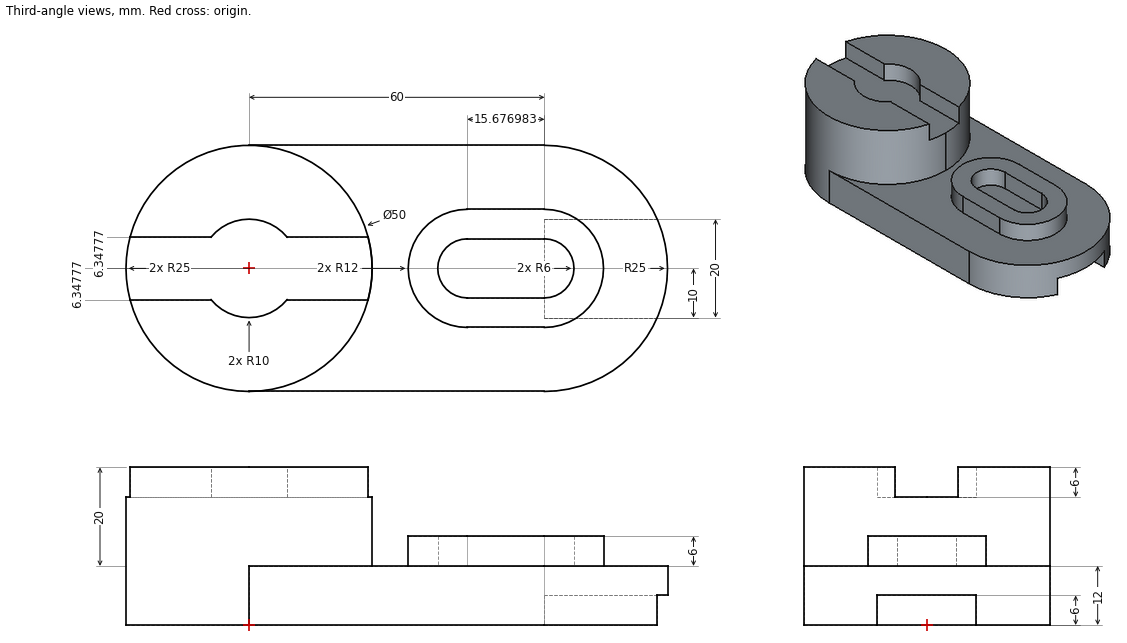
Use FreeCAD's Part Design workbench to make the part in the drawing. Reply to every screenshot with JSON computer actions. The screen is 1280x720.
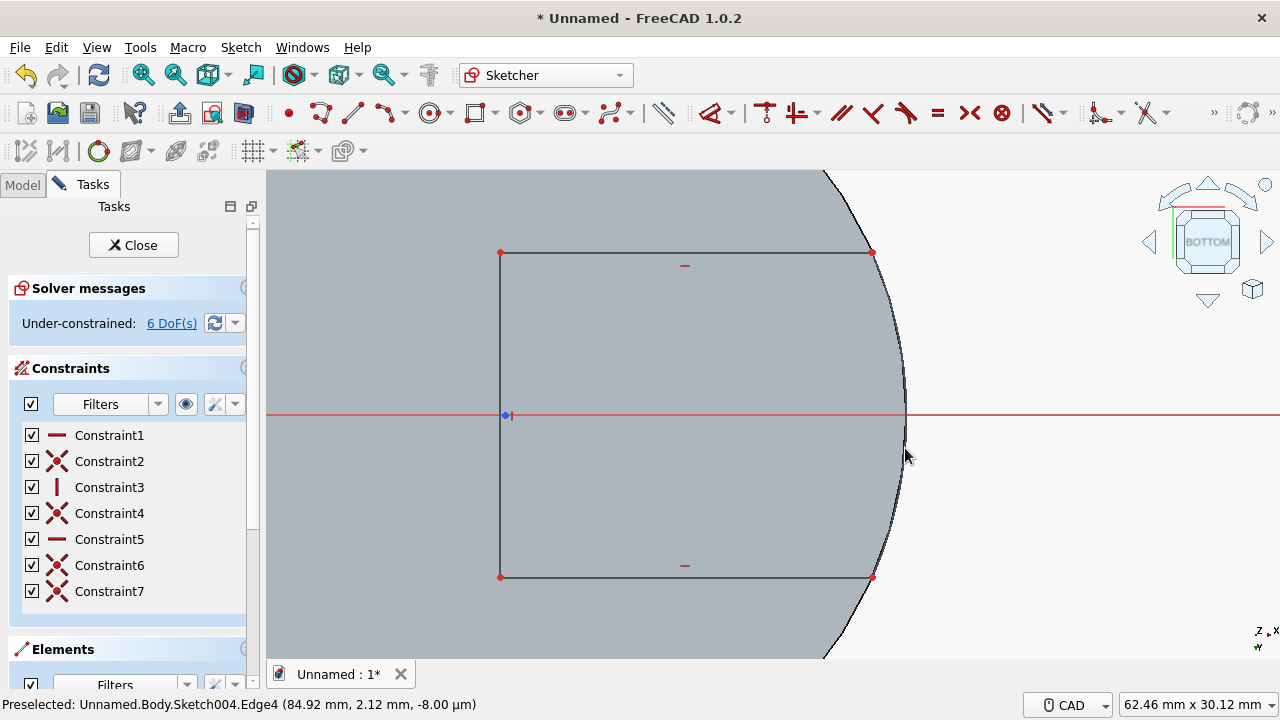
{"action": "left_click", "coordinate": [505, 416]}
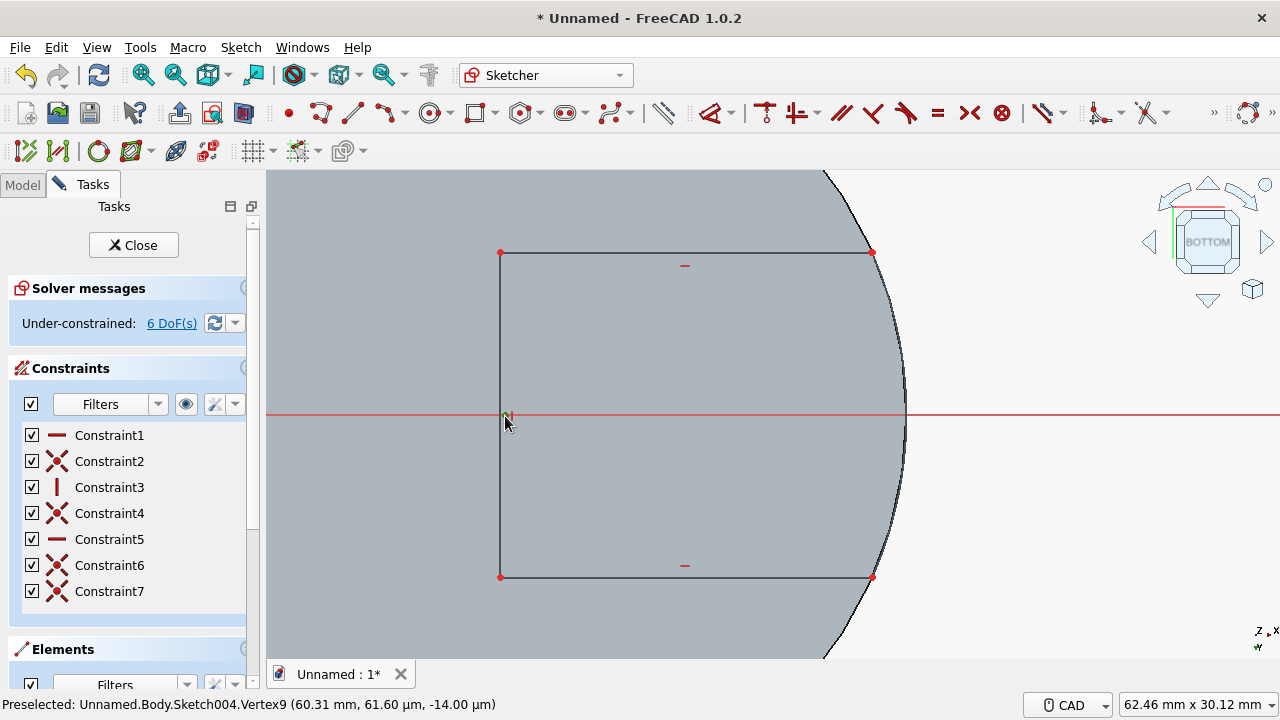
{"action": "left_click", "coordinate": [353, 414]}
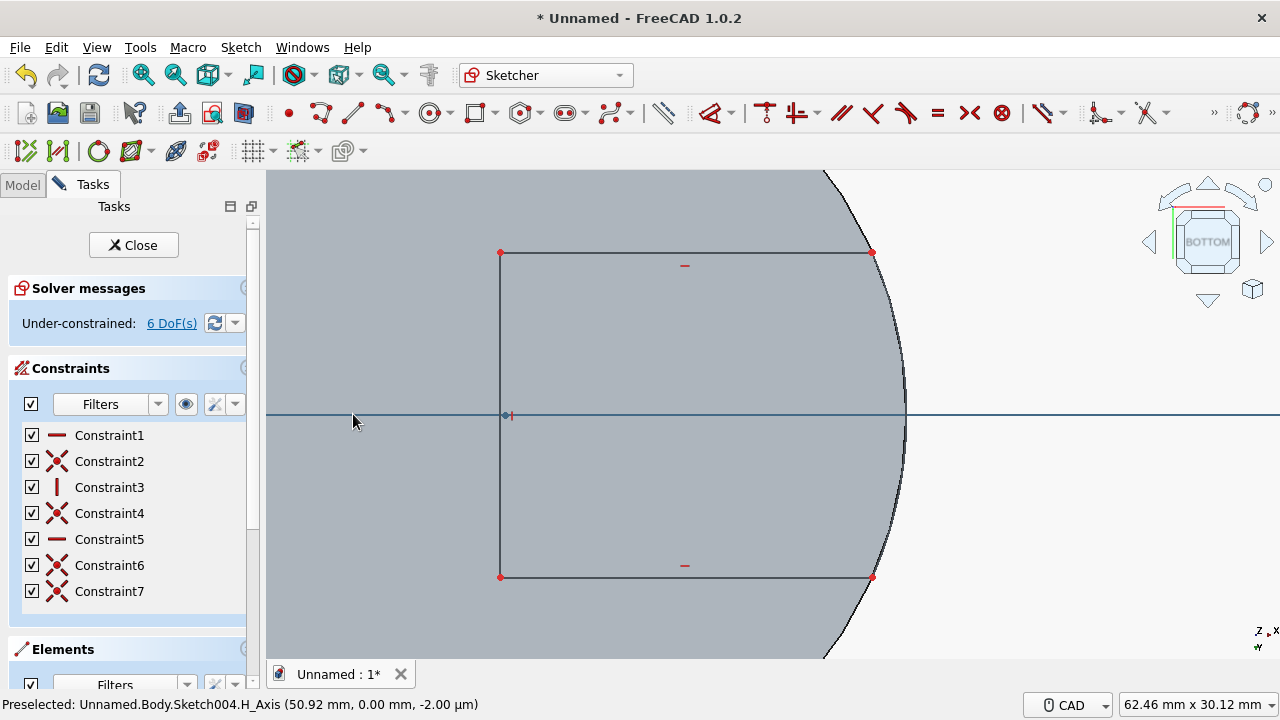
{"action": "left_click", "coordinate": [766, 114]}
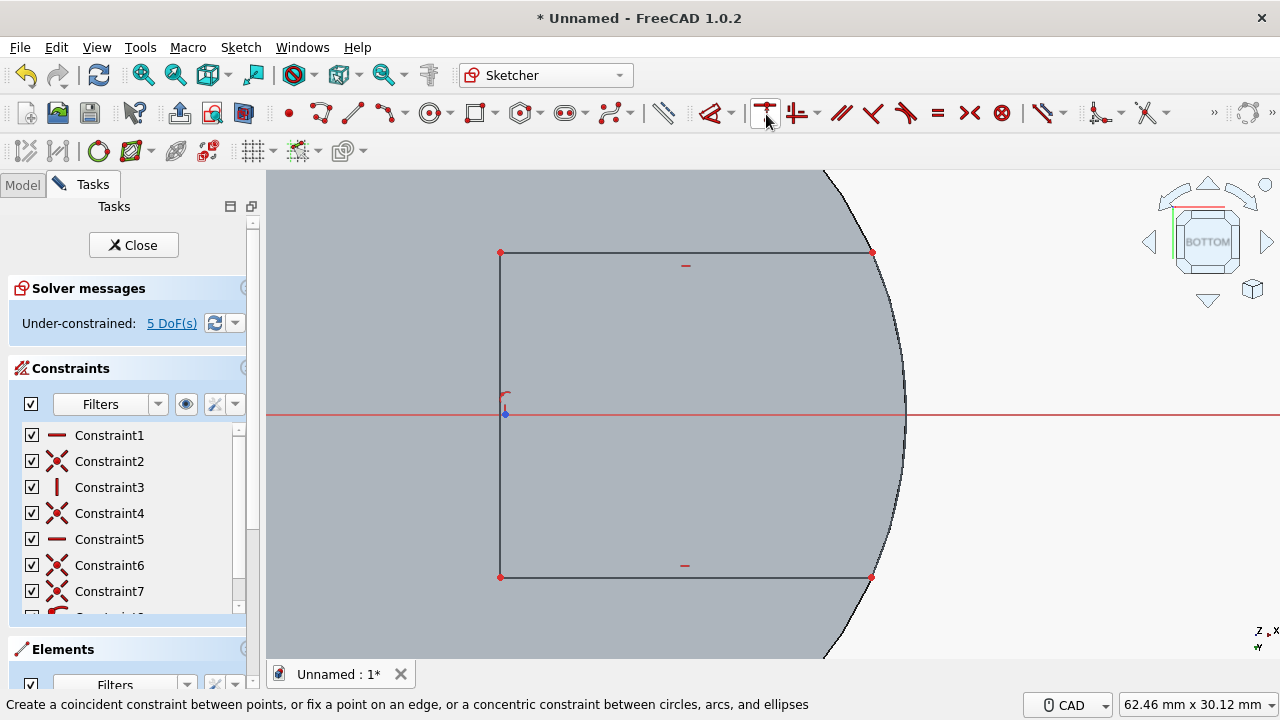
{"action": "key", "text": "d"}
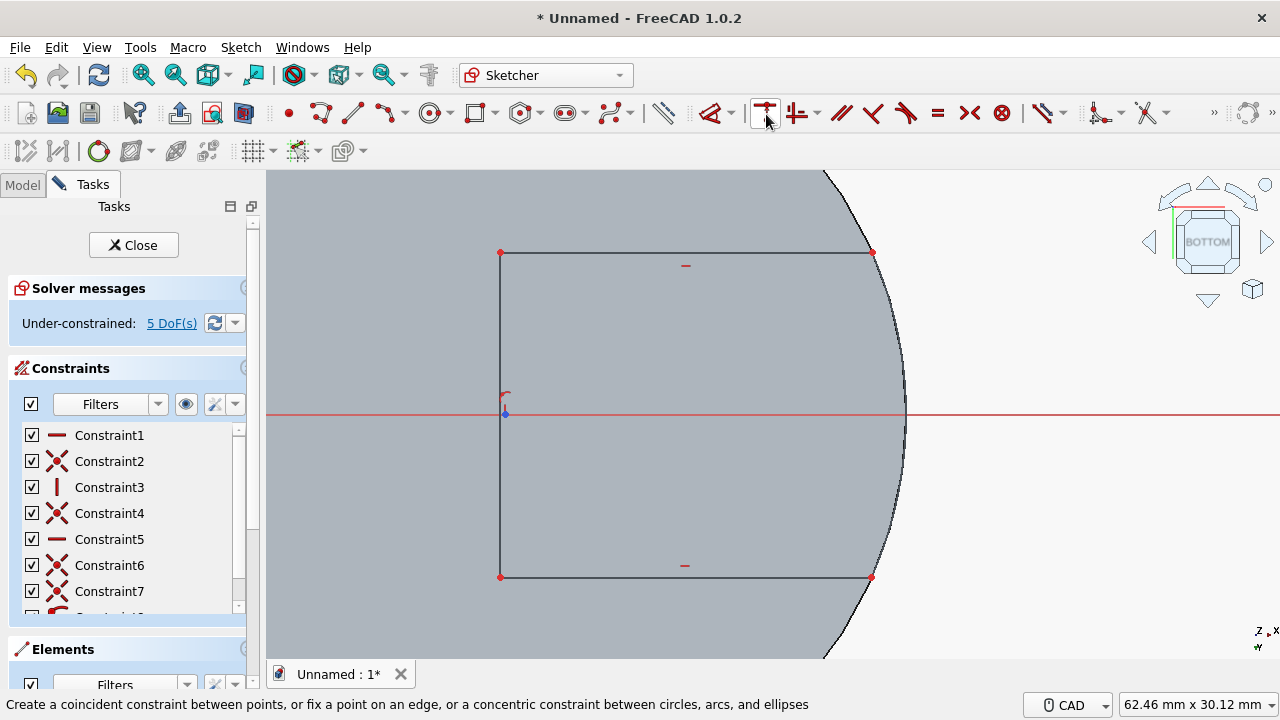
{"action": "left_click", "coordinate": [900, 482]}
{"action": "left_click", "coordinate": [932, 487]}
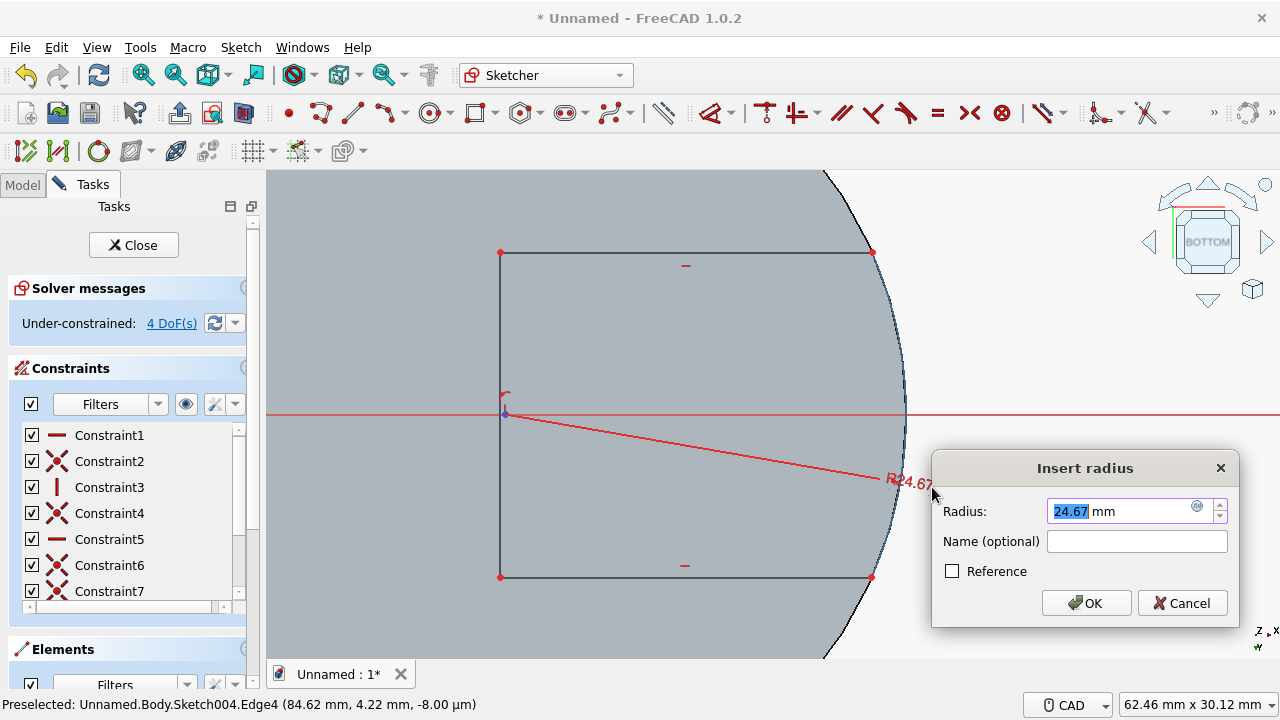
{"action": "type", "text": "25"}
{"action": "key", "text": "Return"}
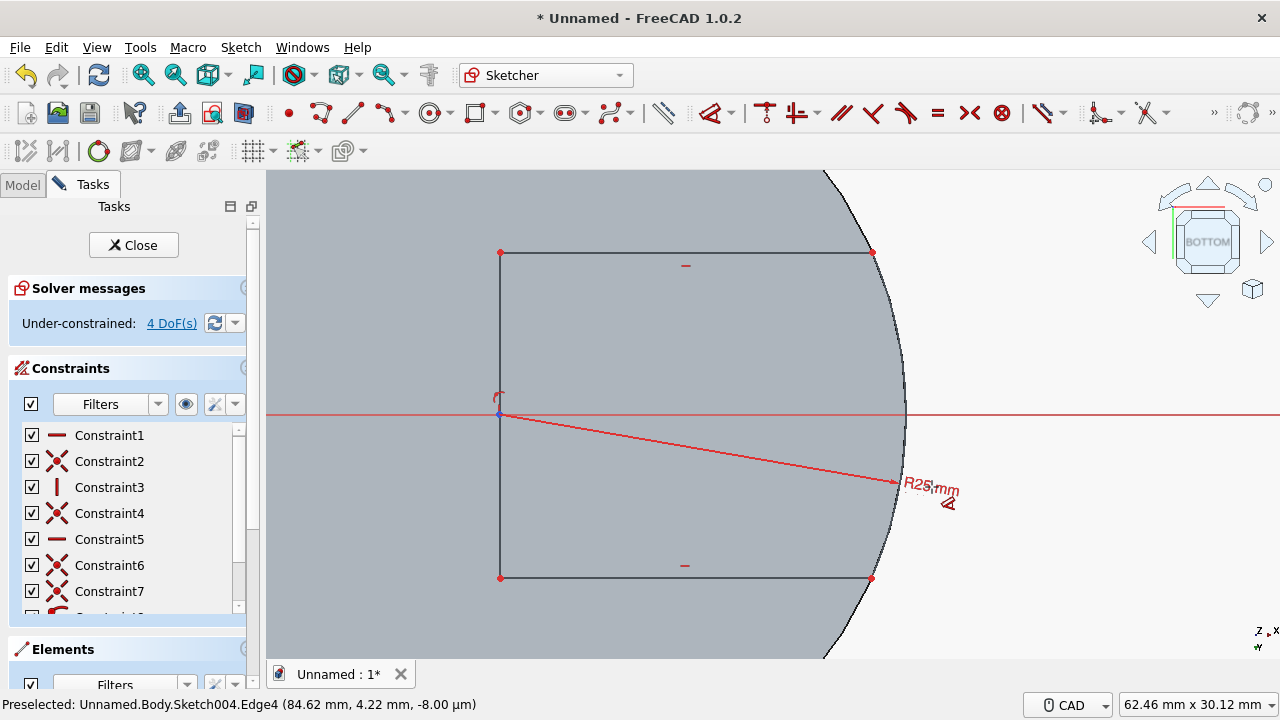
{"action": "left_click", "coordinate": [500, 350]}
{"action": "left_click", "coordinate": [466, 341]}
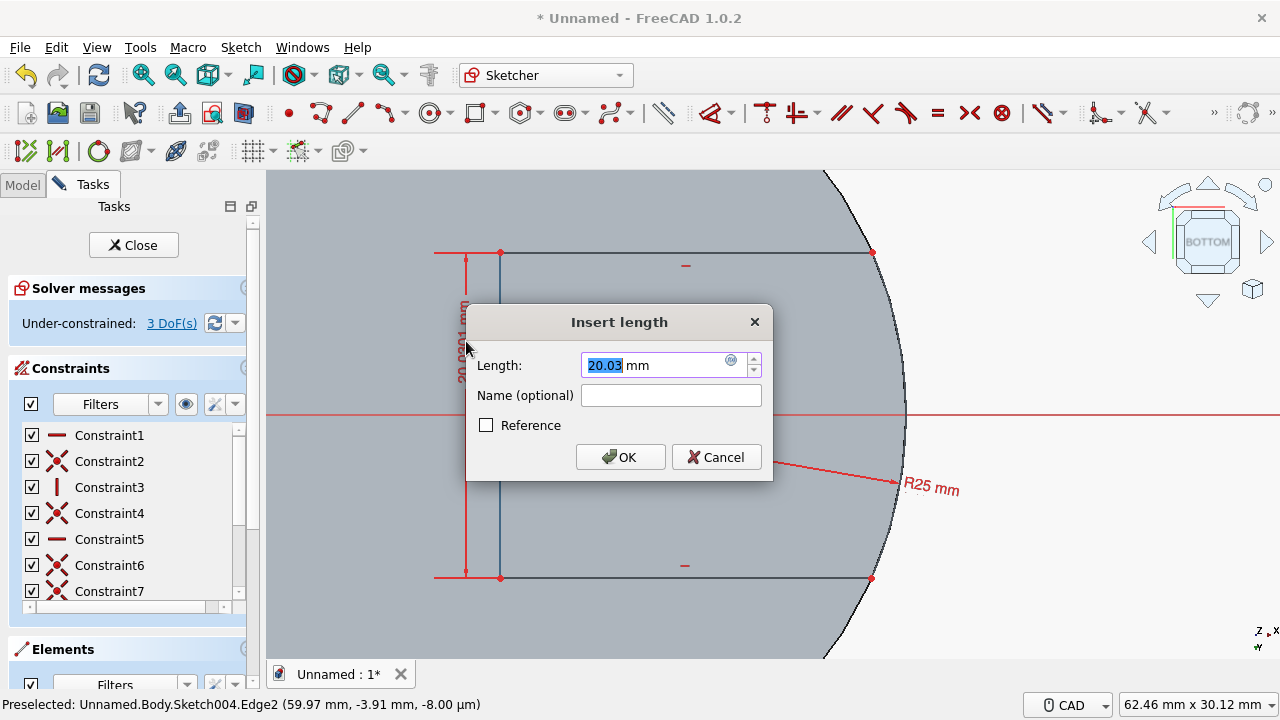
{"action": "type", "text": "20"}
{"action": "key", "text": "Return"}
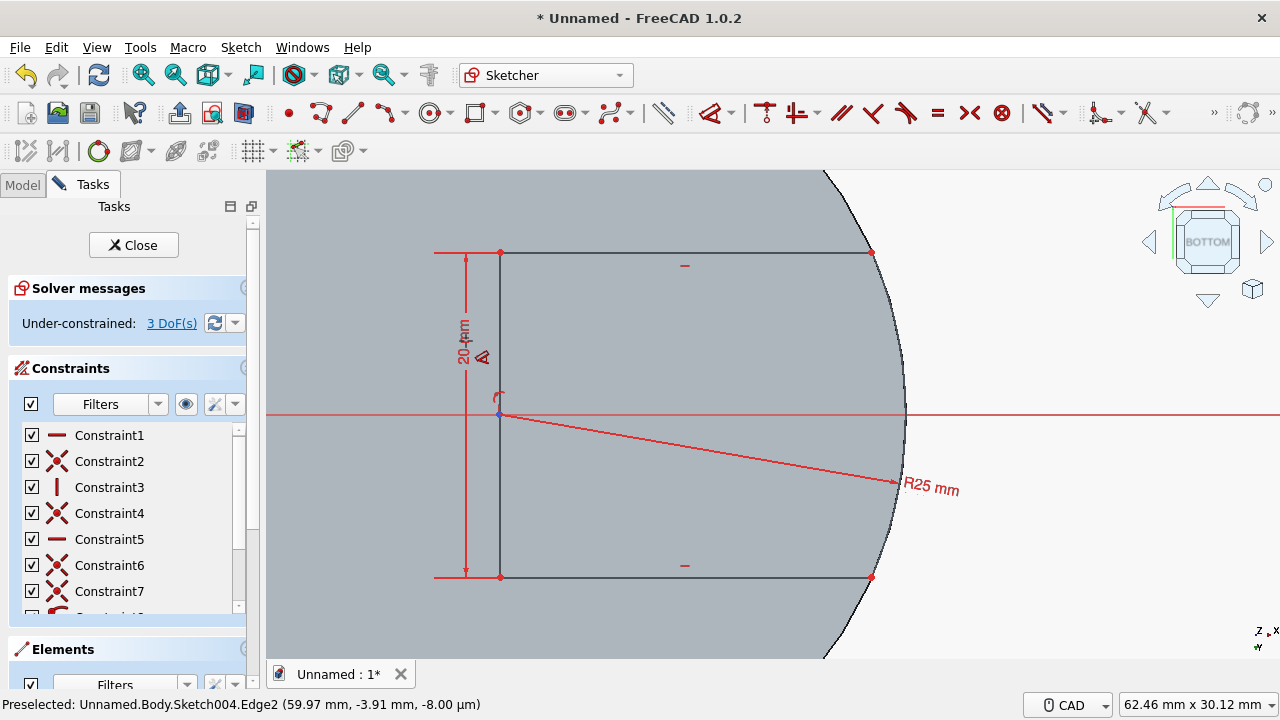
{"action": "left_click", "coordinate": [872, 253]}
{"action": "left_click", "coordinate": [906, 297]}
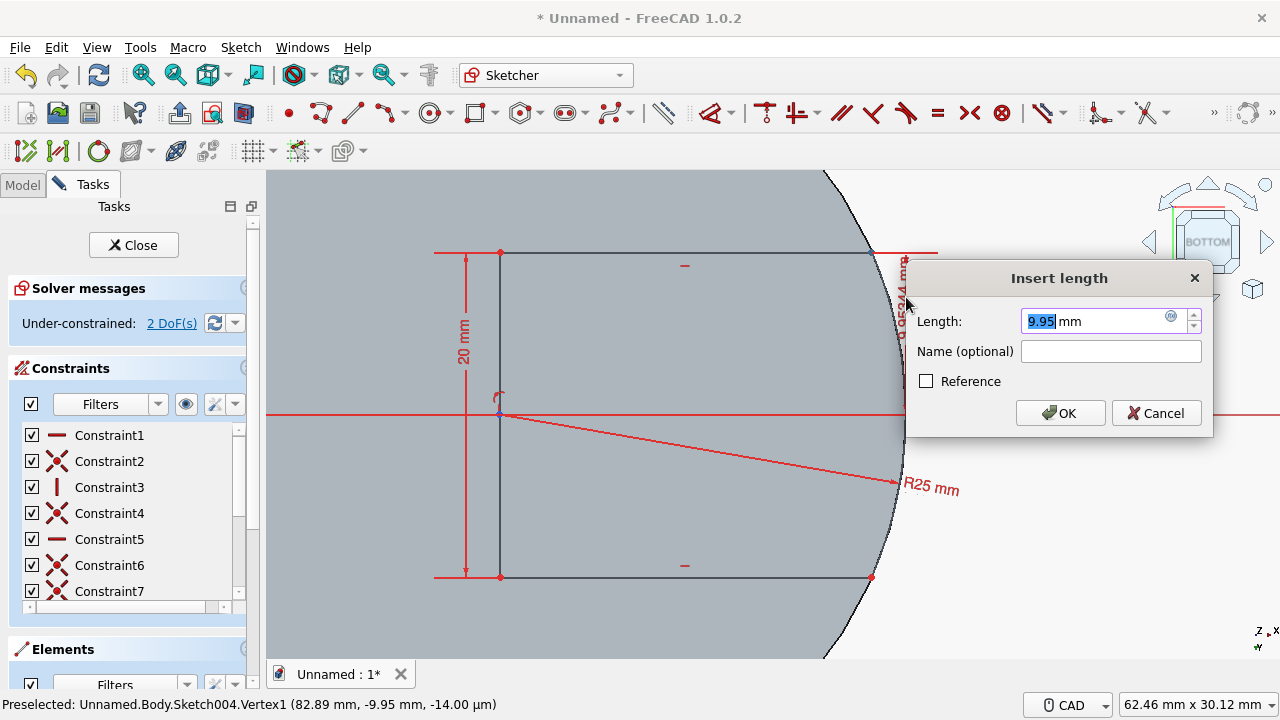
{"action": "type", "text": "10"}
{"action": "key", "text": "Return"}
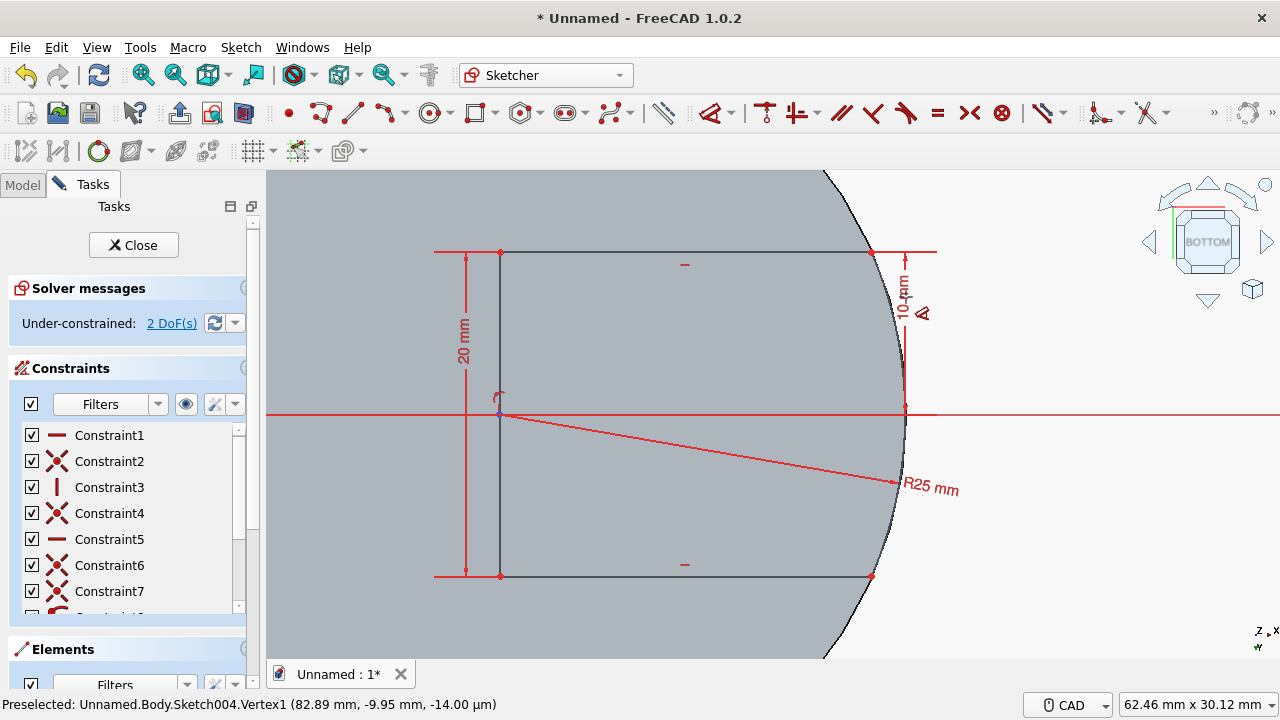
{"action": "left_click", "coordinate": [500, 252]}
{"action": "left_click", "coordinate": [397, 218]}